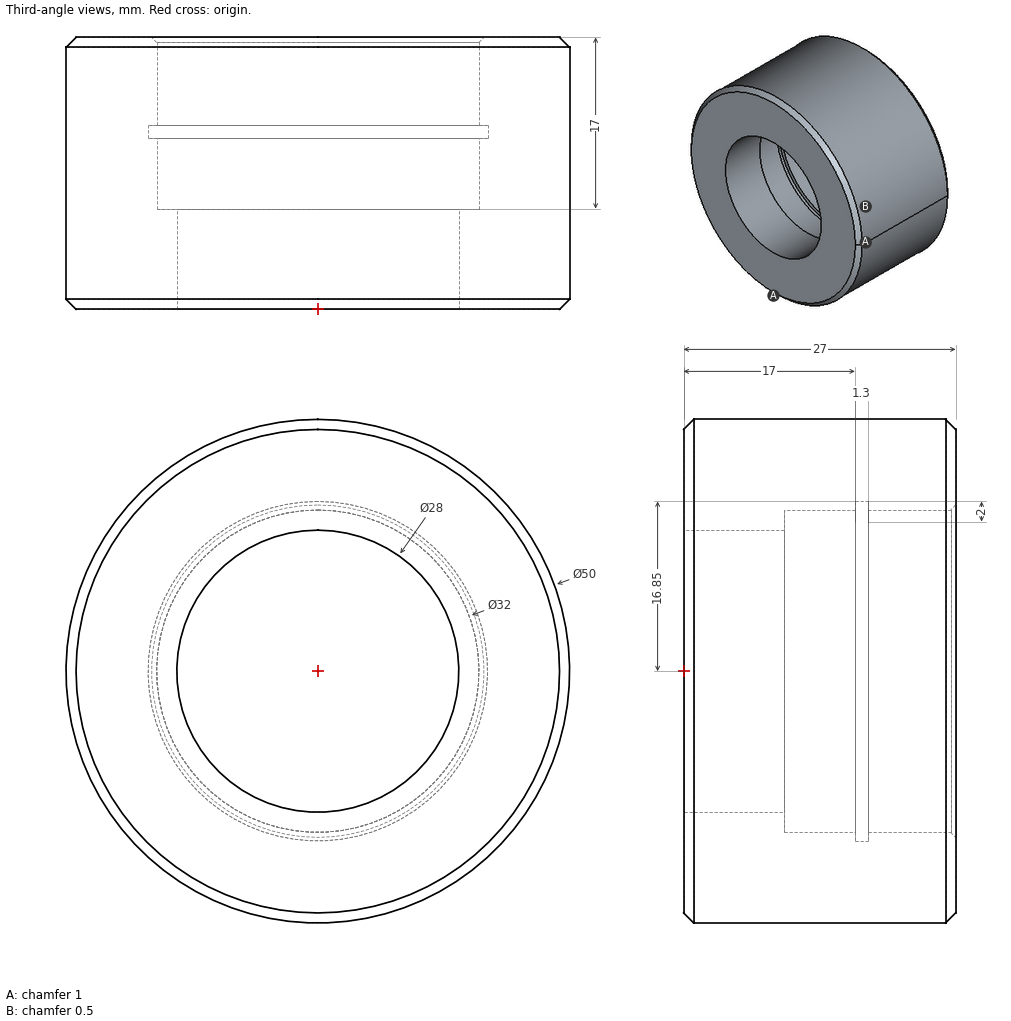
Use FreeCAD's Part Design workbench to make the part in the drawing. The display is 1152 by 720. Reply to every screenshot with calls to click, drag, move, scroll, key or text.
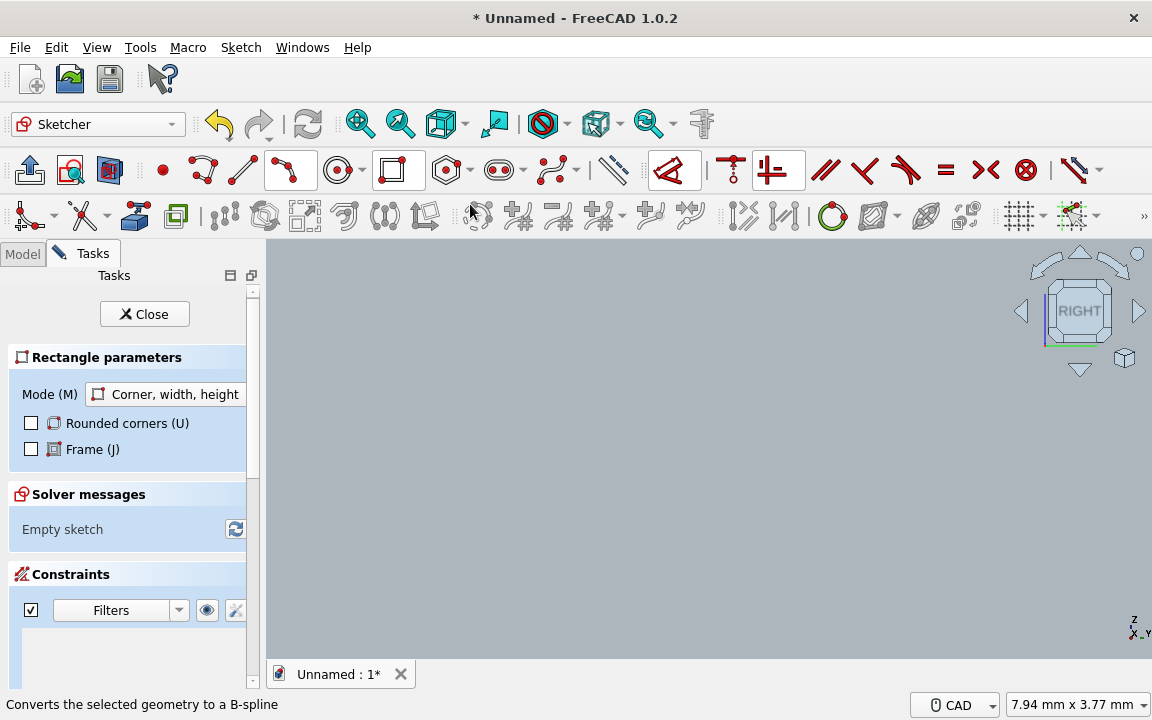
click(555, 339)
move(700, 562)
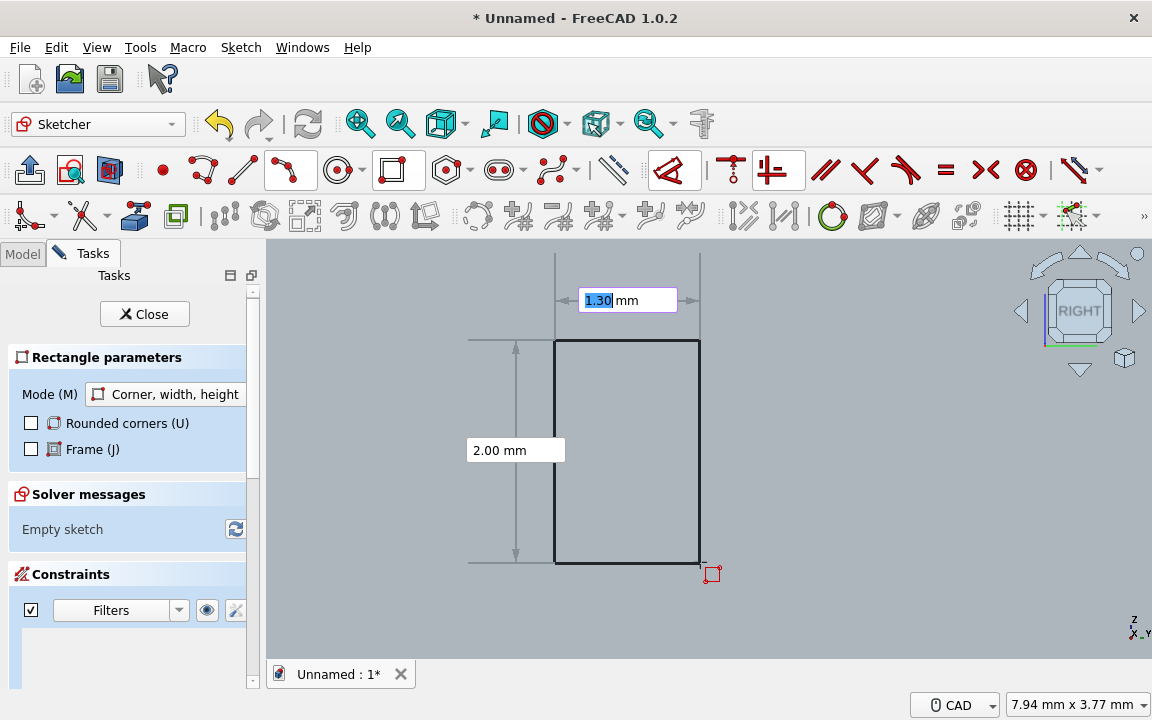
text(1.3)
key(Tab)
text(2)
key(Return)
key(Escape)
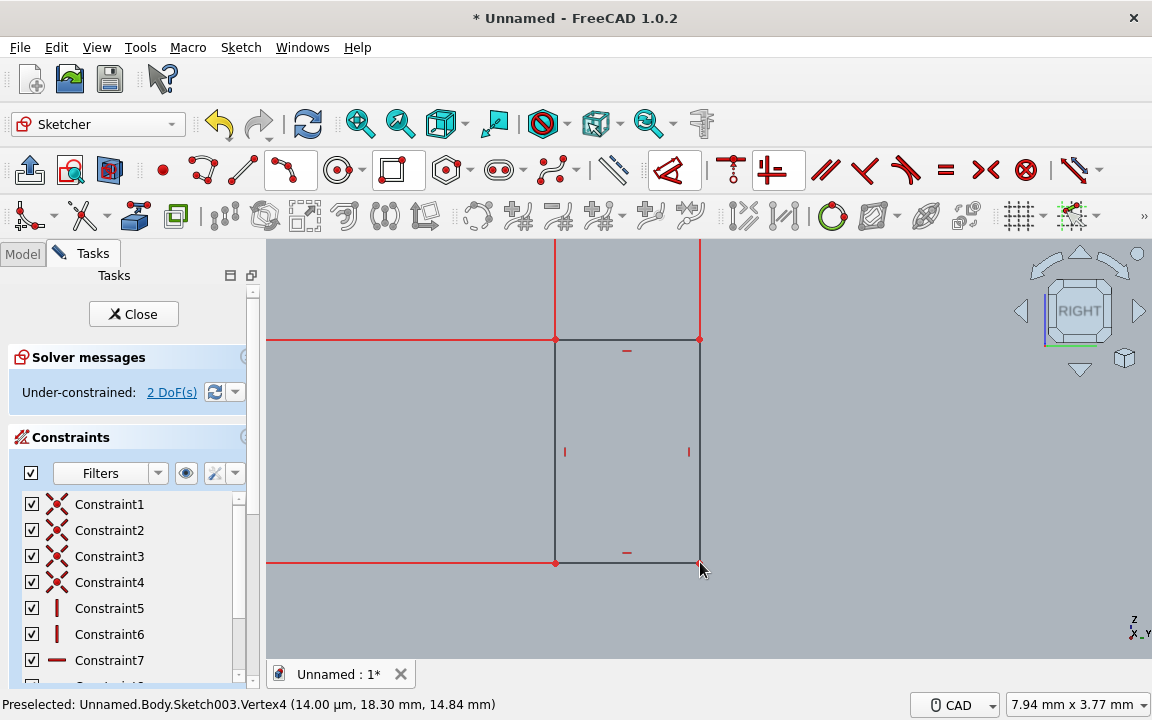
click(668, 170)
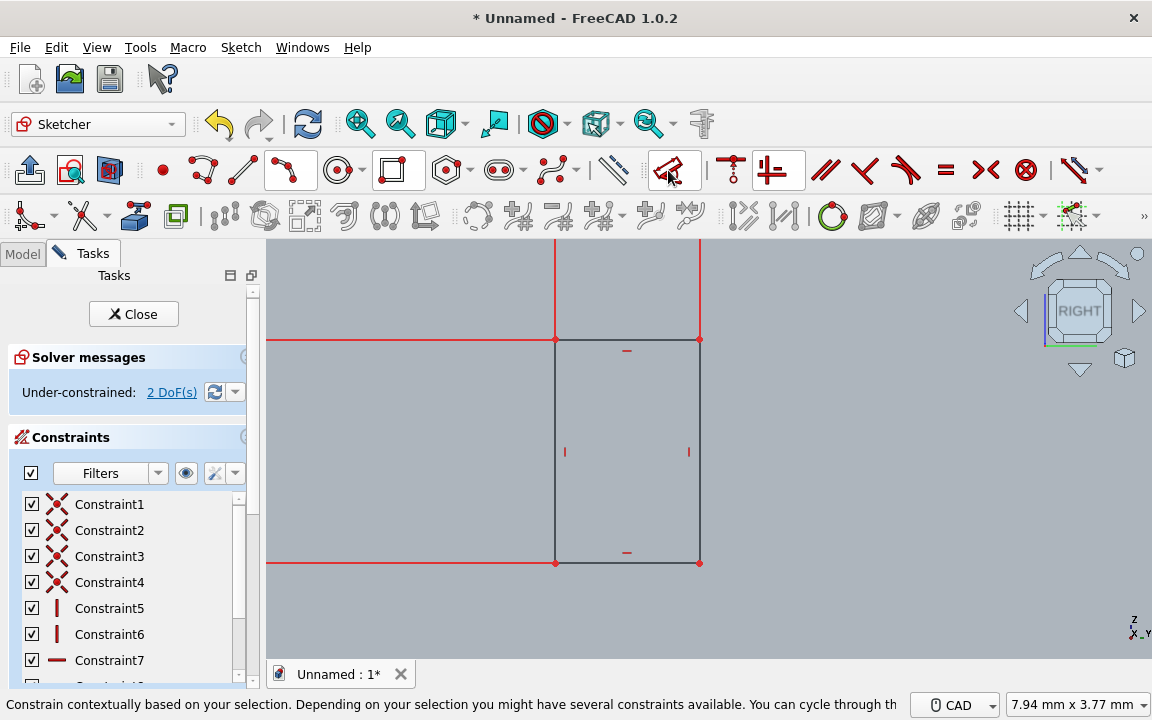
click(555, 340)
click(425, 306)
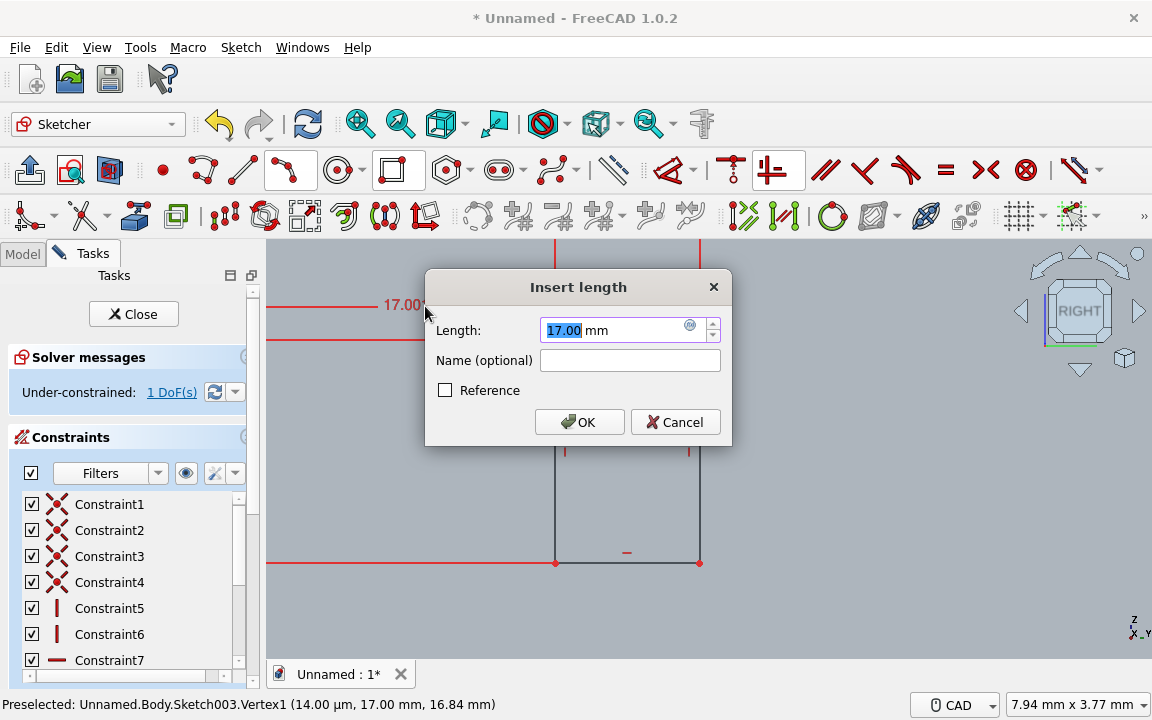
text(17)
key(Return)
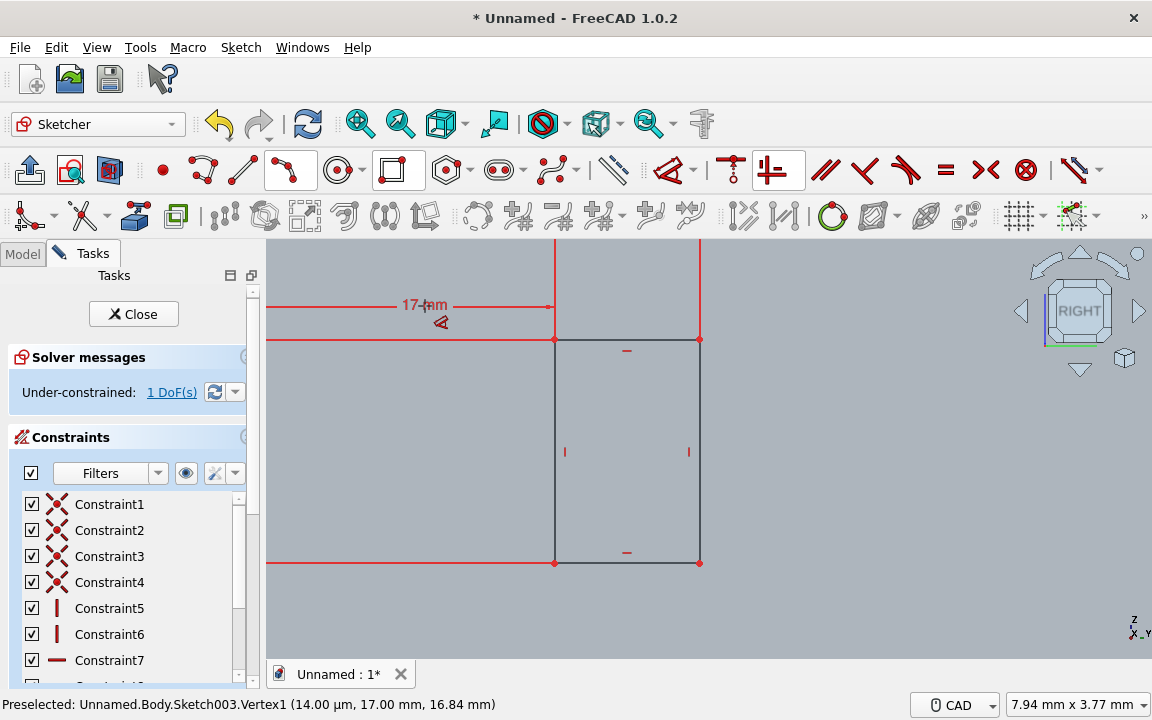
click(555, 340)
click(589, 485)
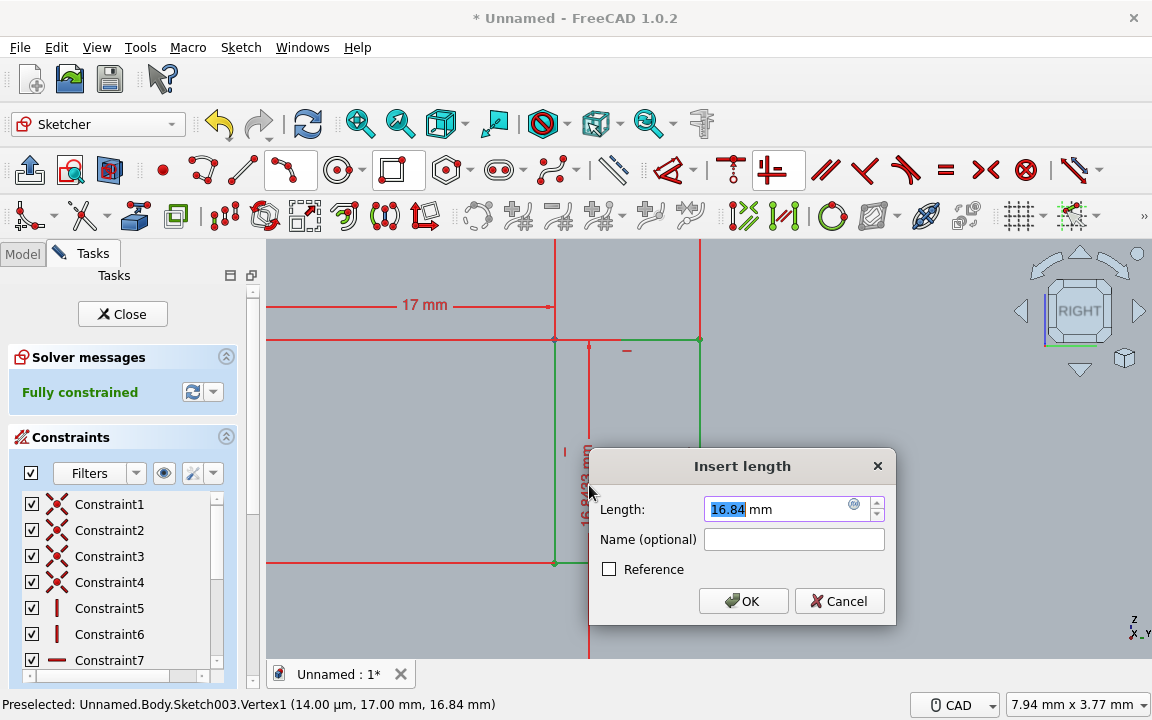
text(16.85)
key(Return)
key(Escape)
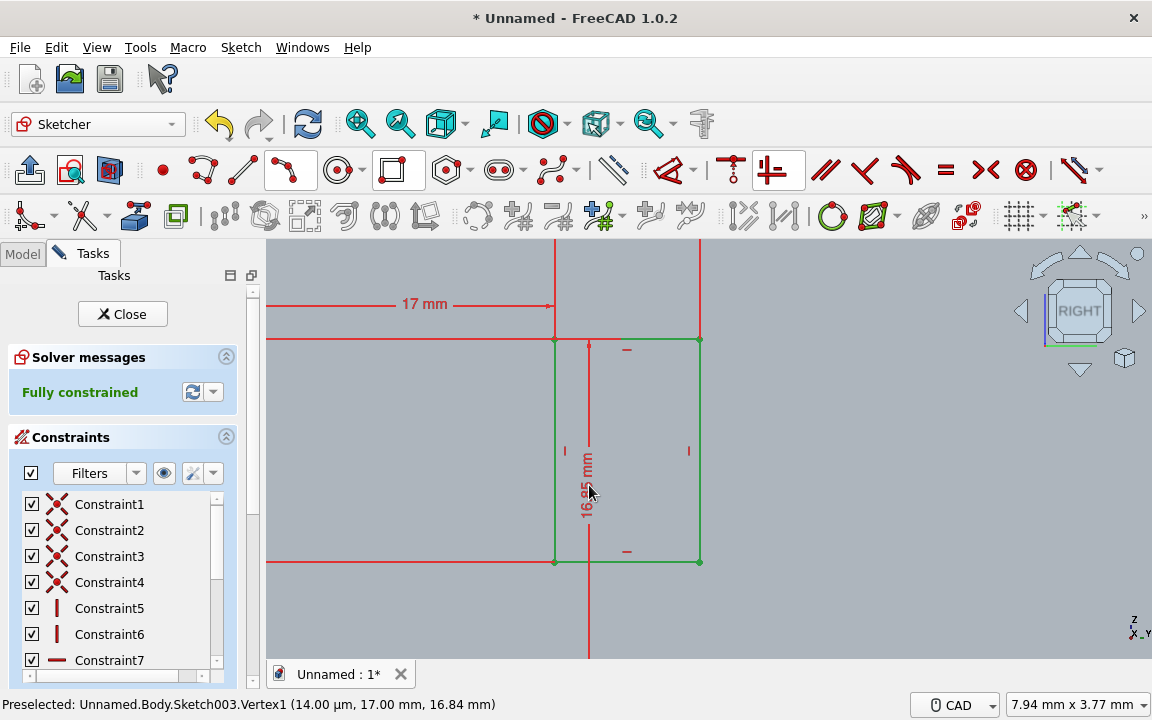
click(123, 314)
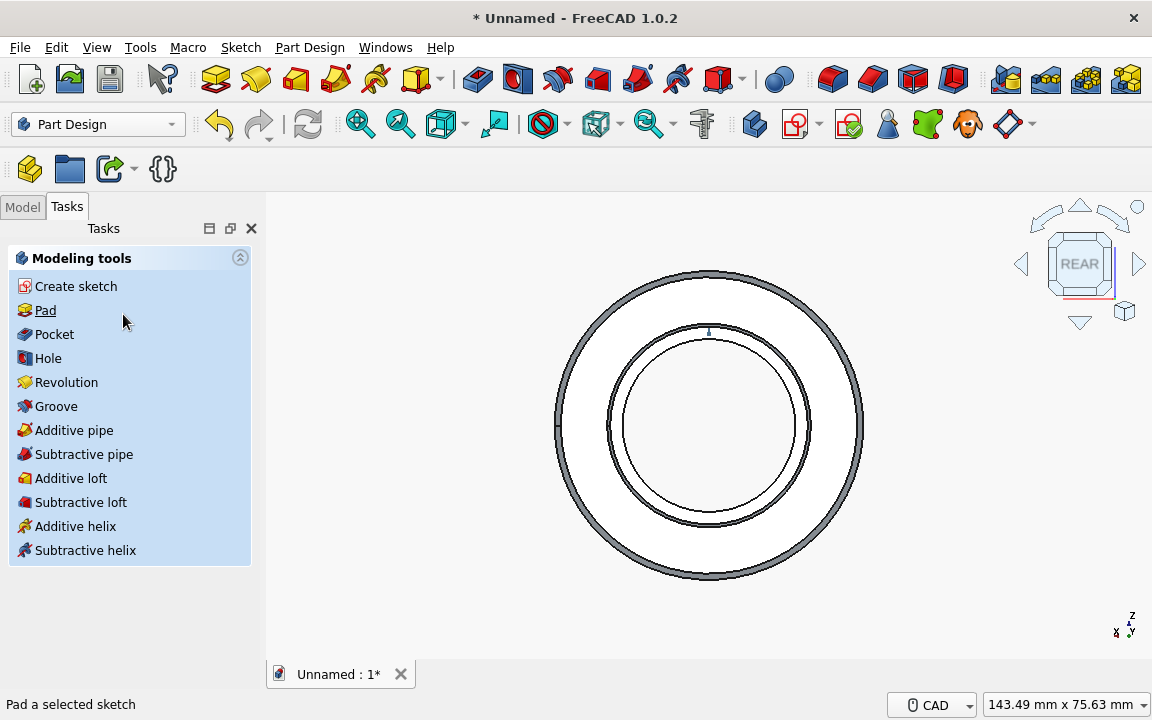
click(558, 80)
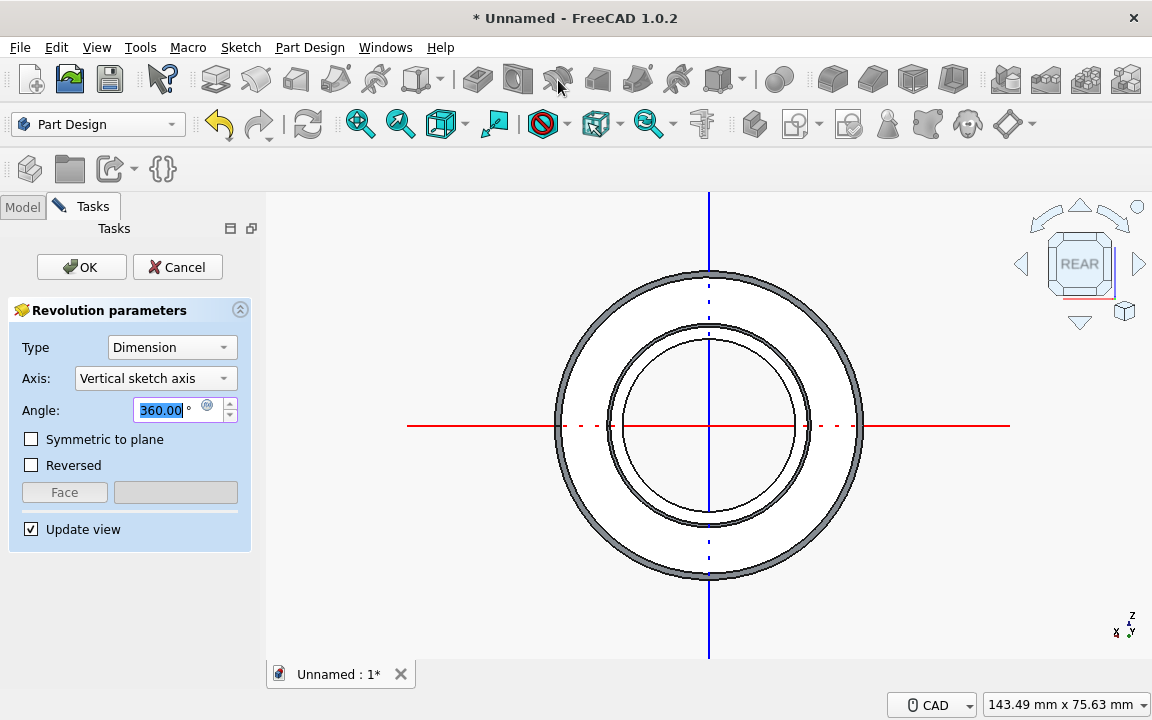
click(156, 378)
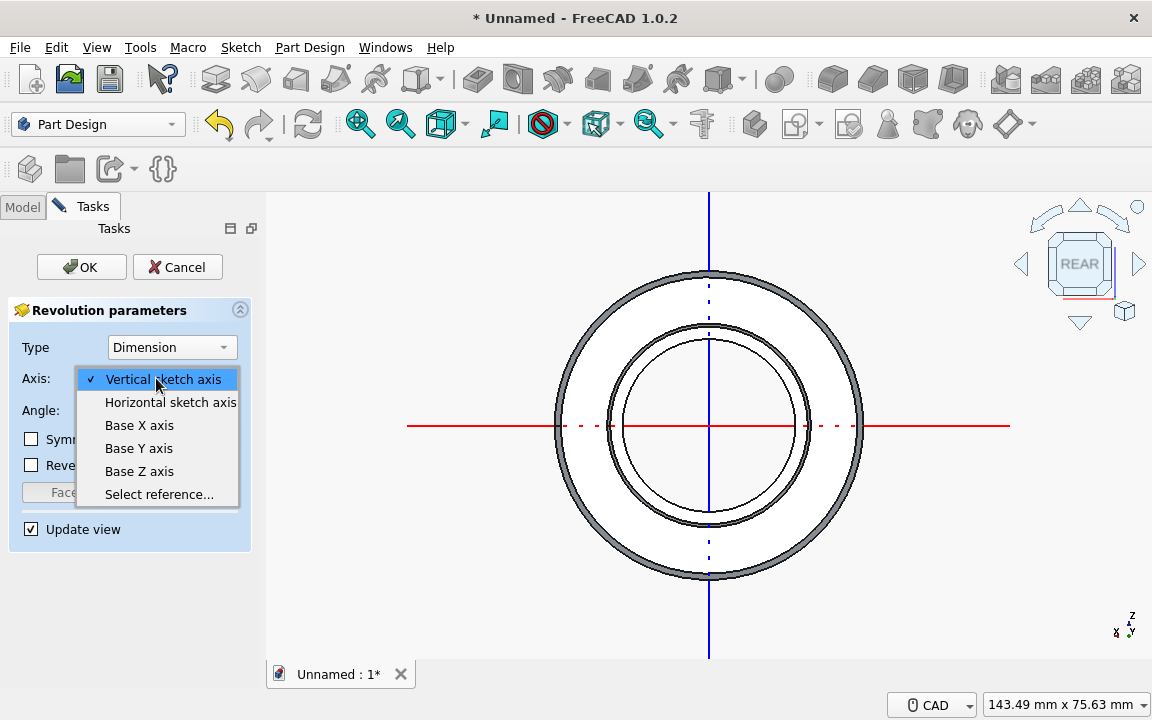
click(156, 402)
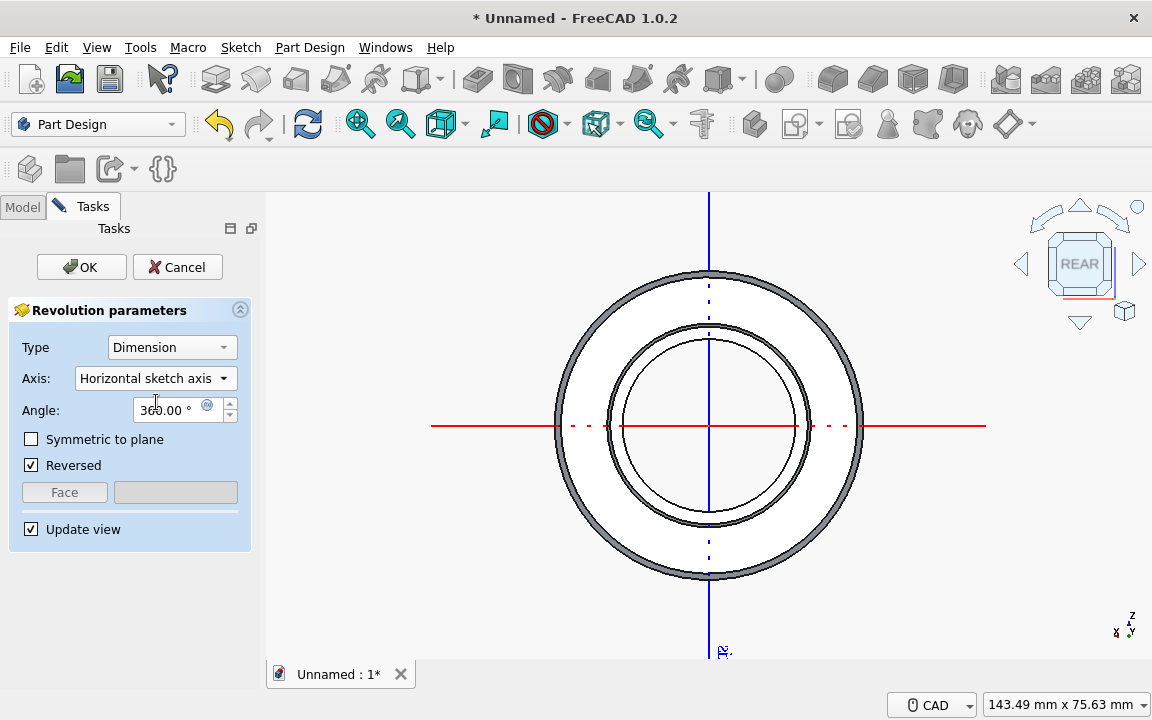
click(82, 267)